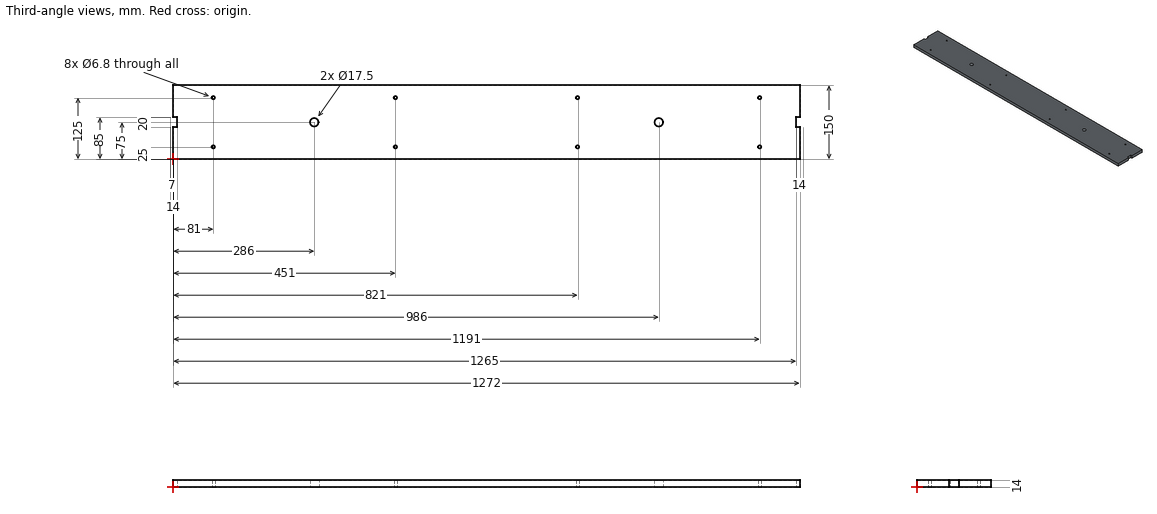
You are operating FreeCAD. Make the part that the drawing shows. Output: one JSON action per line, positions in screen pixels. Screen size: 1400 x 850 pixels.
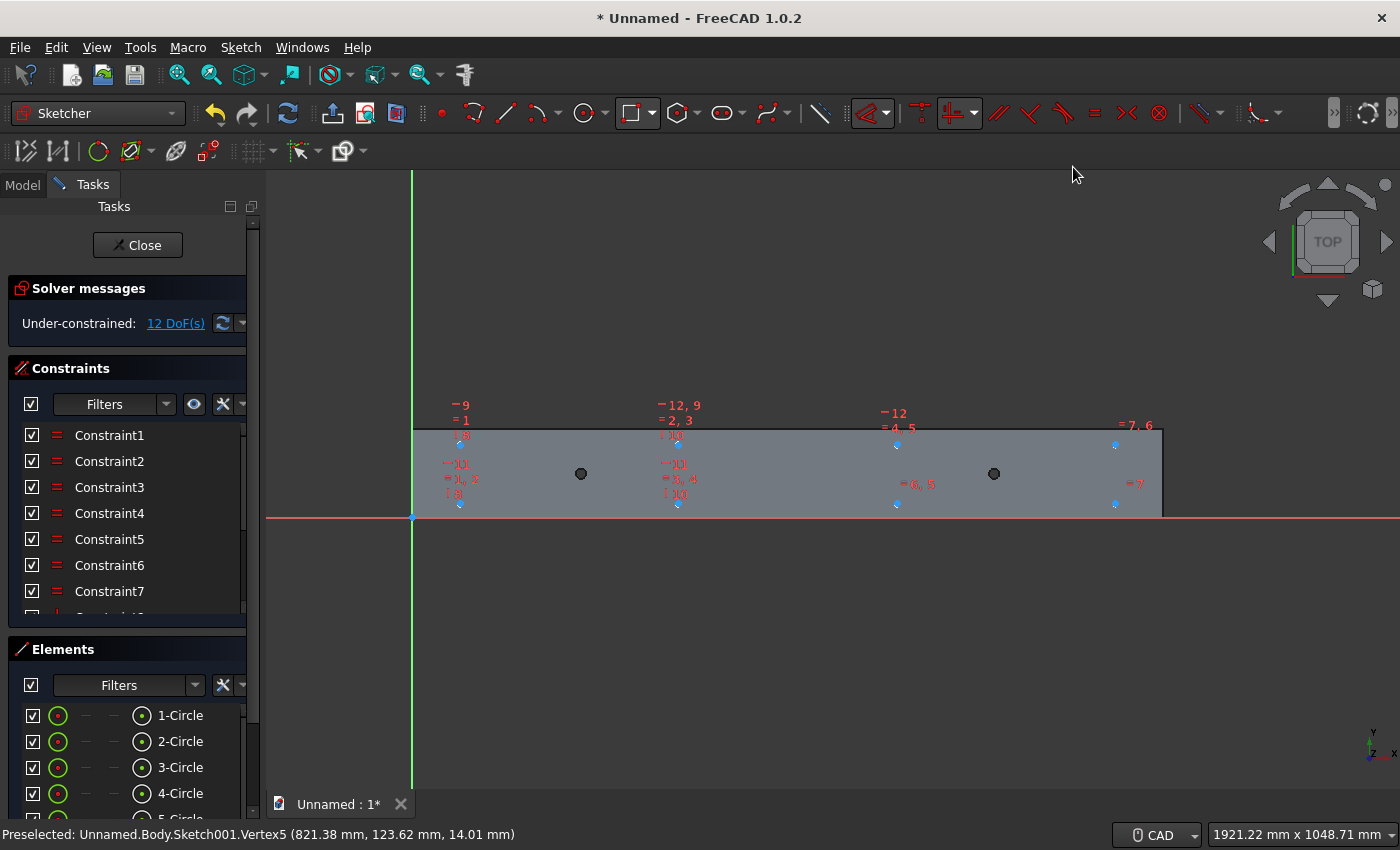
{"action": "left_click", "coordinate": [897, 445]}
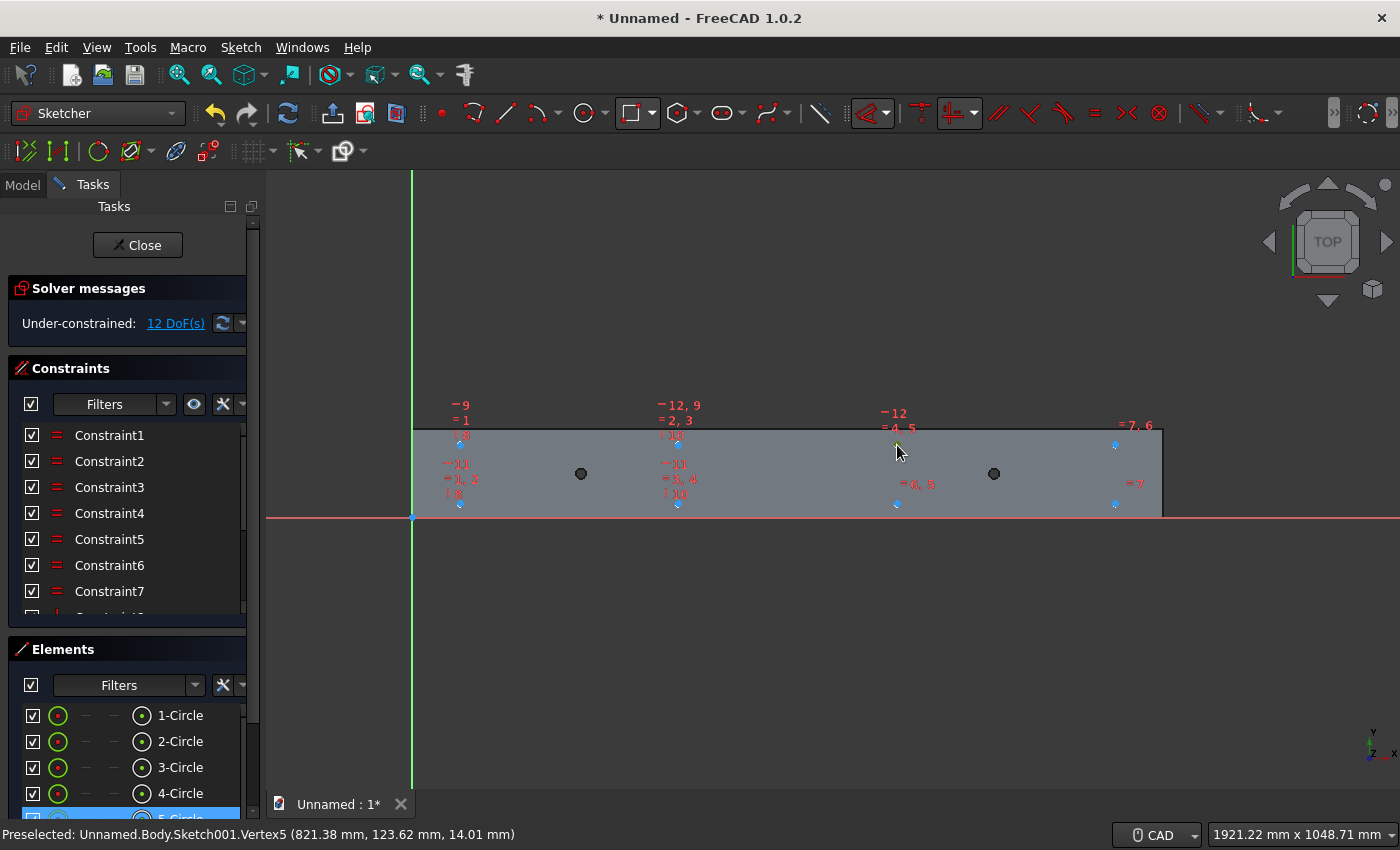
{"action": "left_click", "coordinate": [897, 504]}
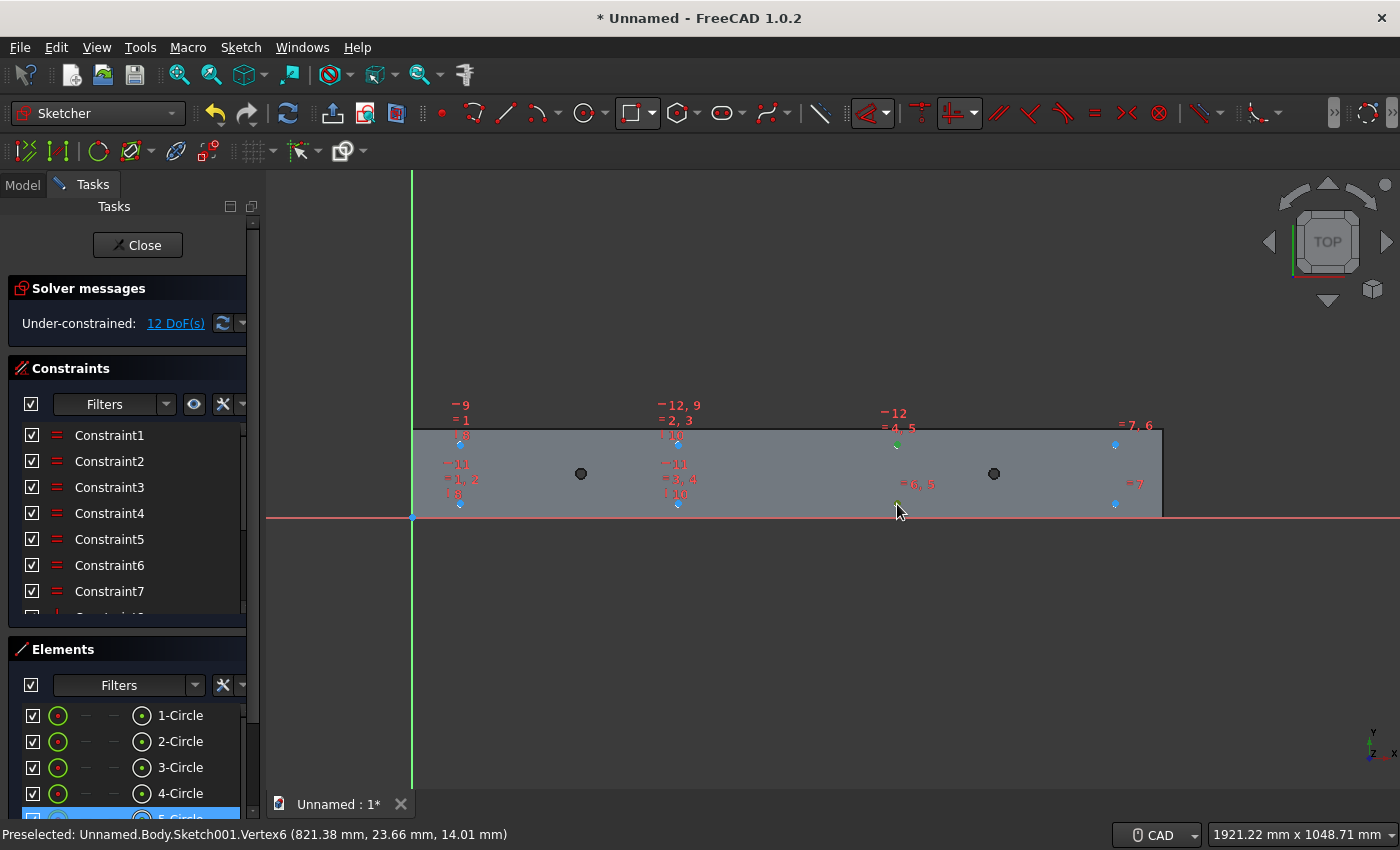
{"action": "key", "text": "v"}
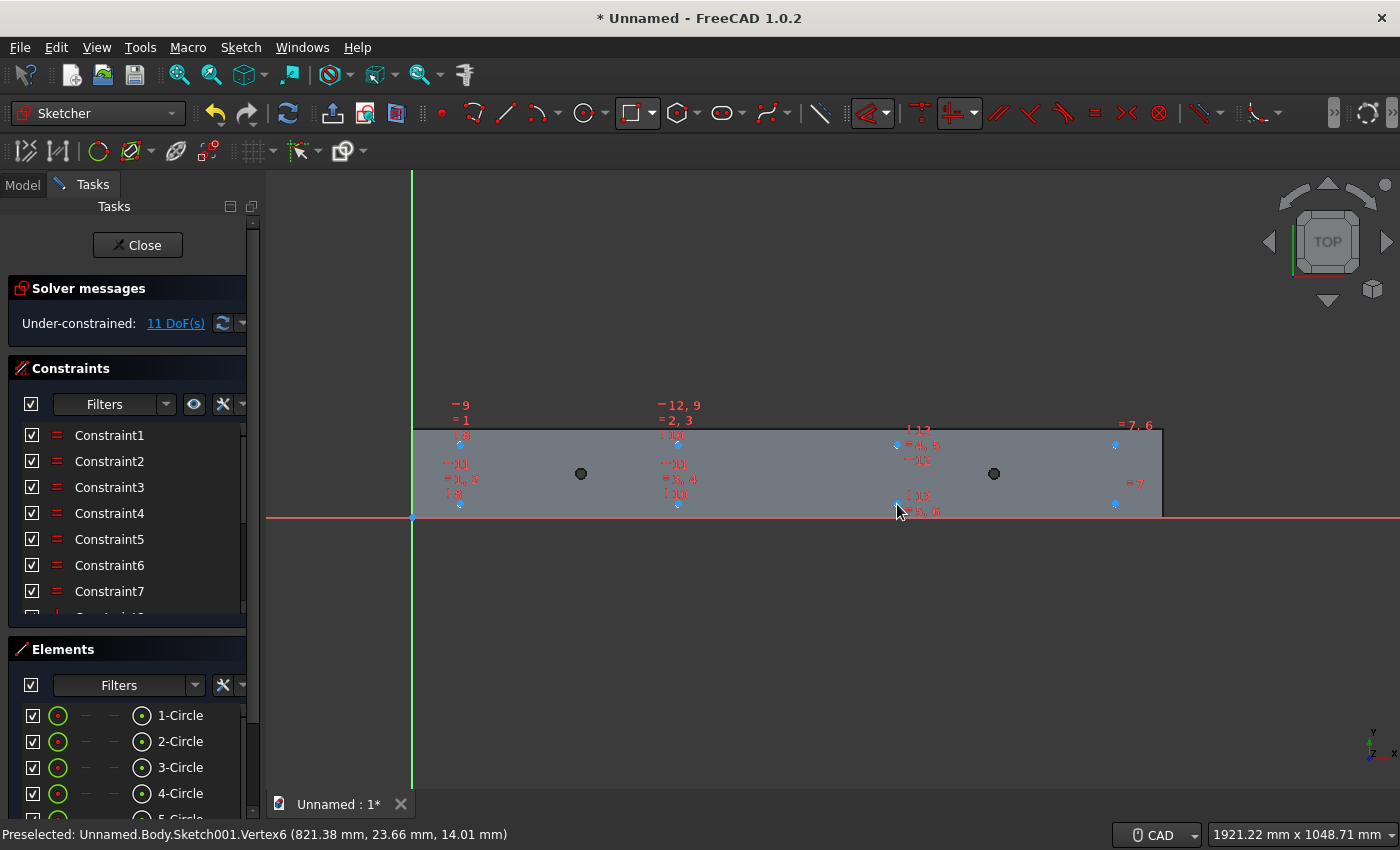
{"action": "left_click", "coordinate": [678, 504]}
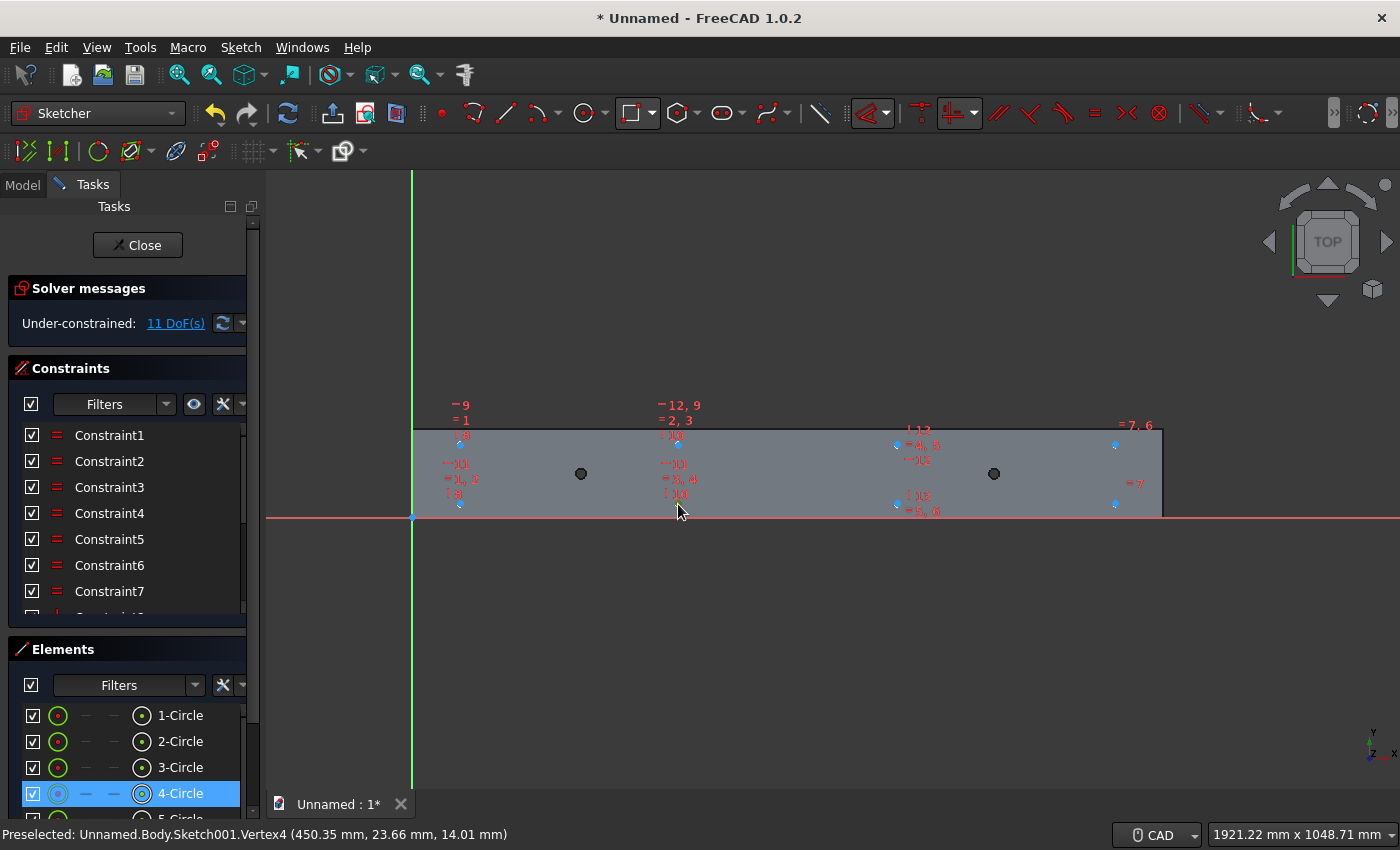
{"action": "left_click", "coordinate": [897, 504]}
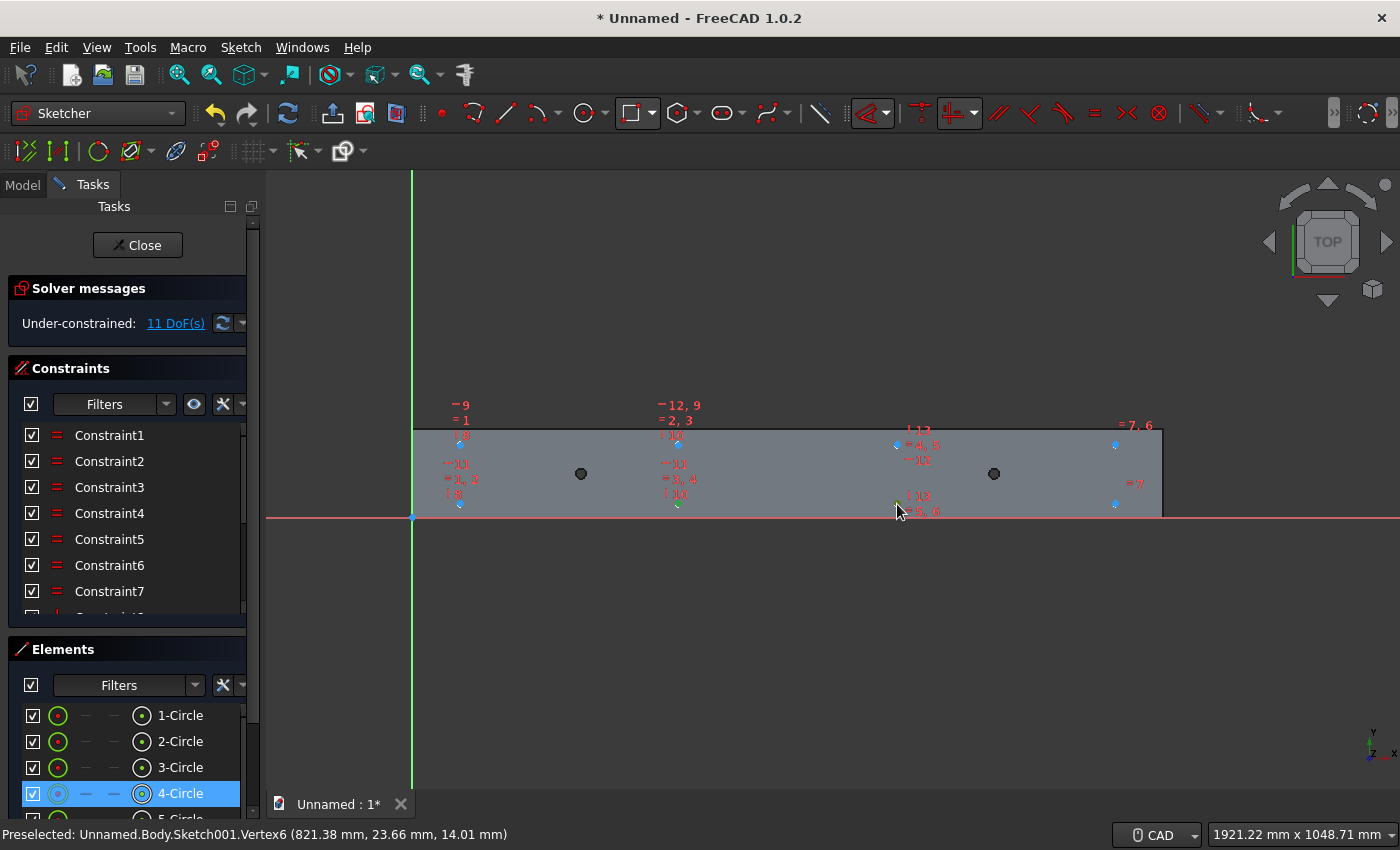
{"action": "left_click", "coordinate": [976, 114]}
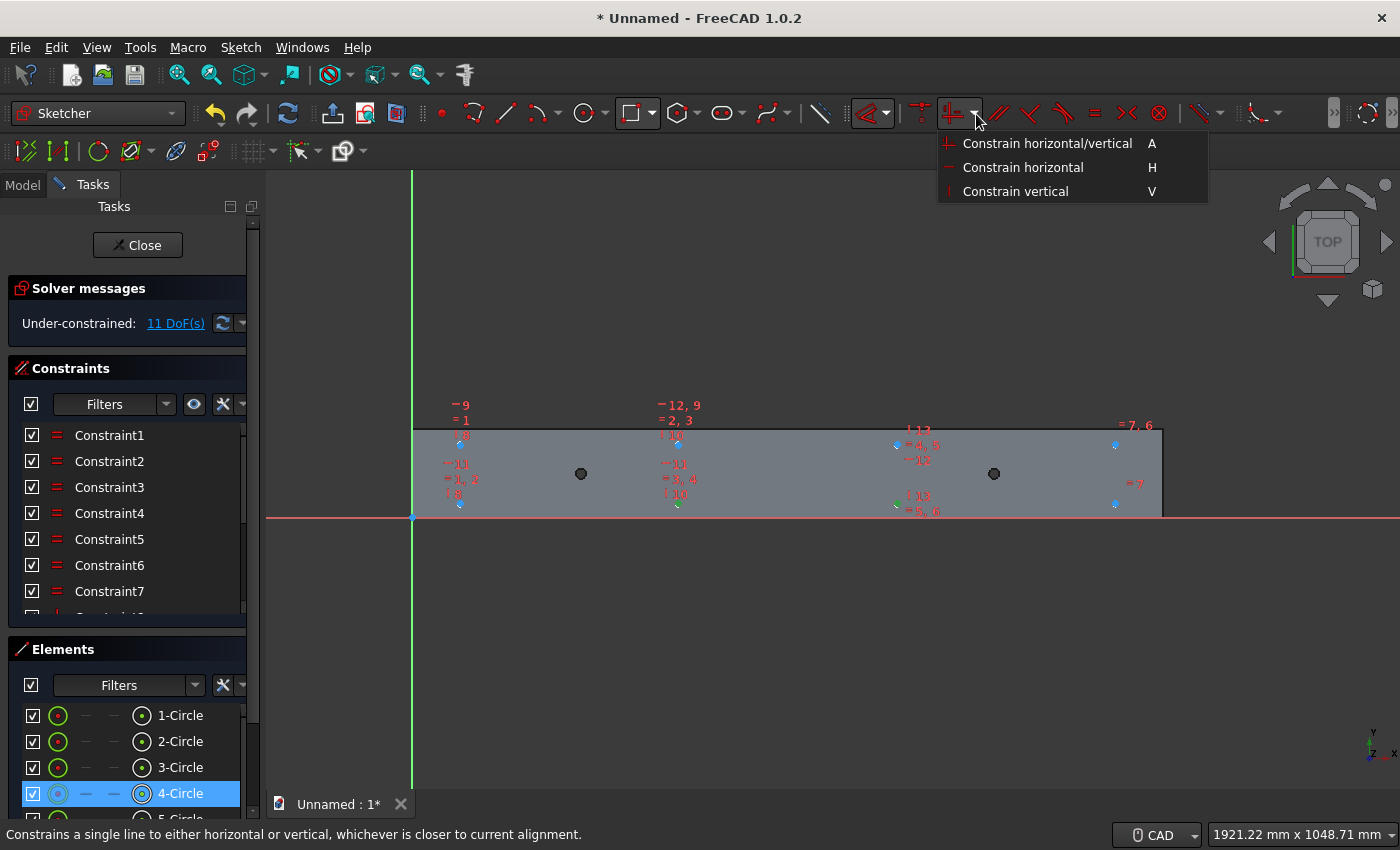
{"action": "left_click", "coordinate": [1073, 167]}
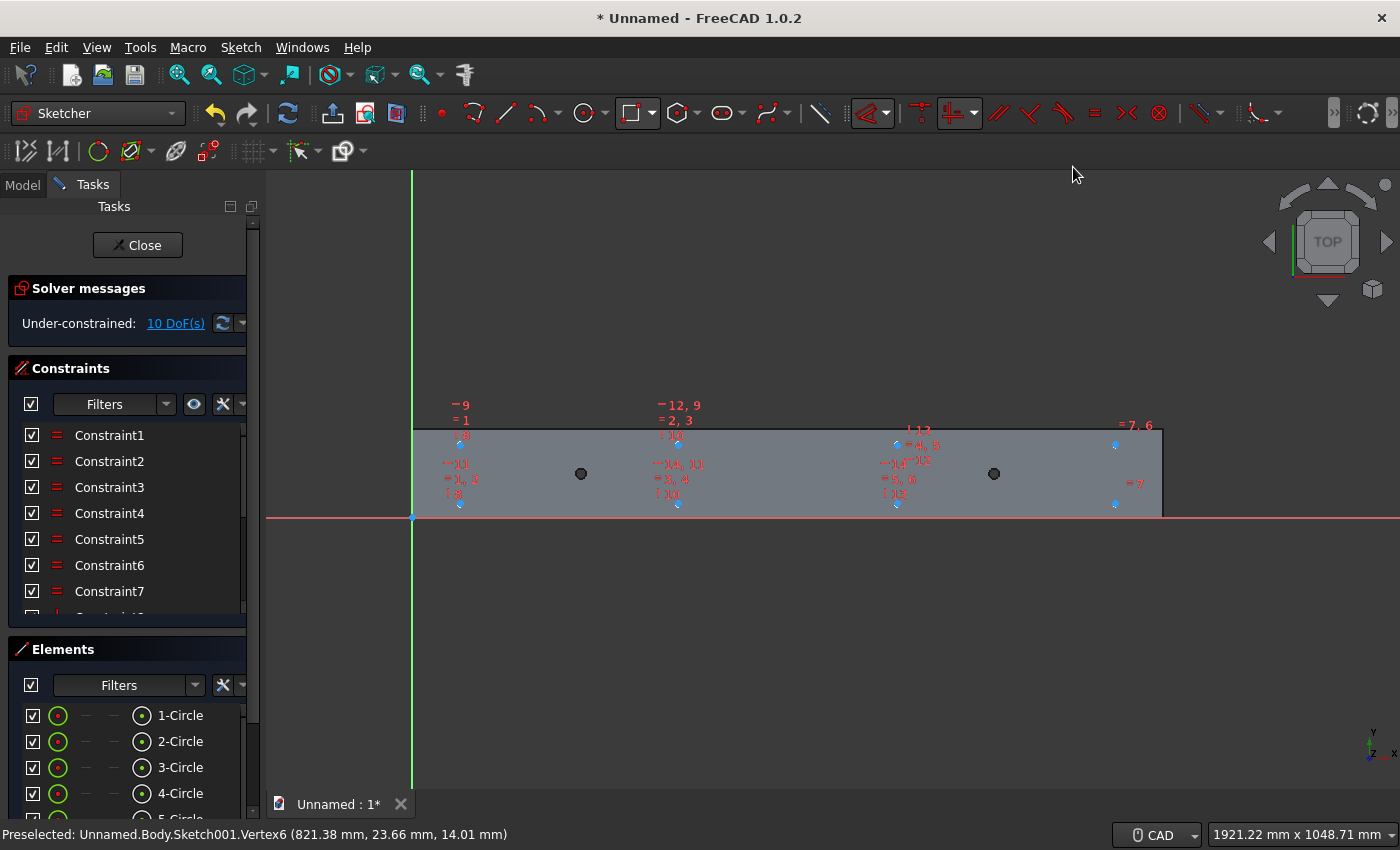
{"action": "left_click", "coordinate": [897, 445]}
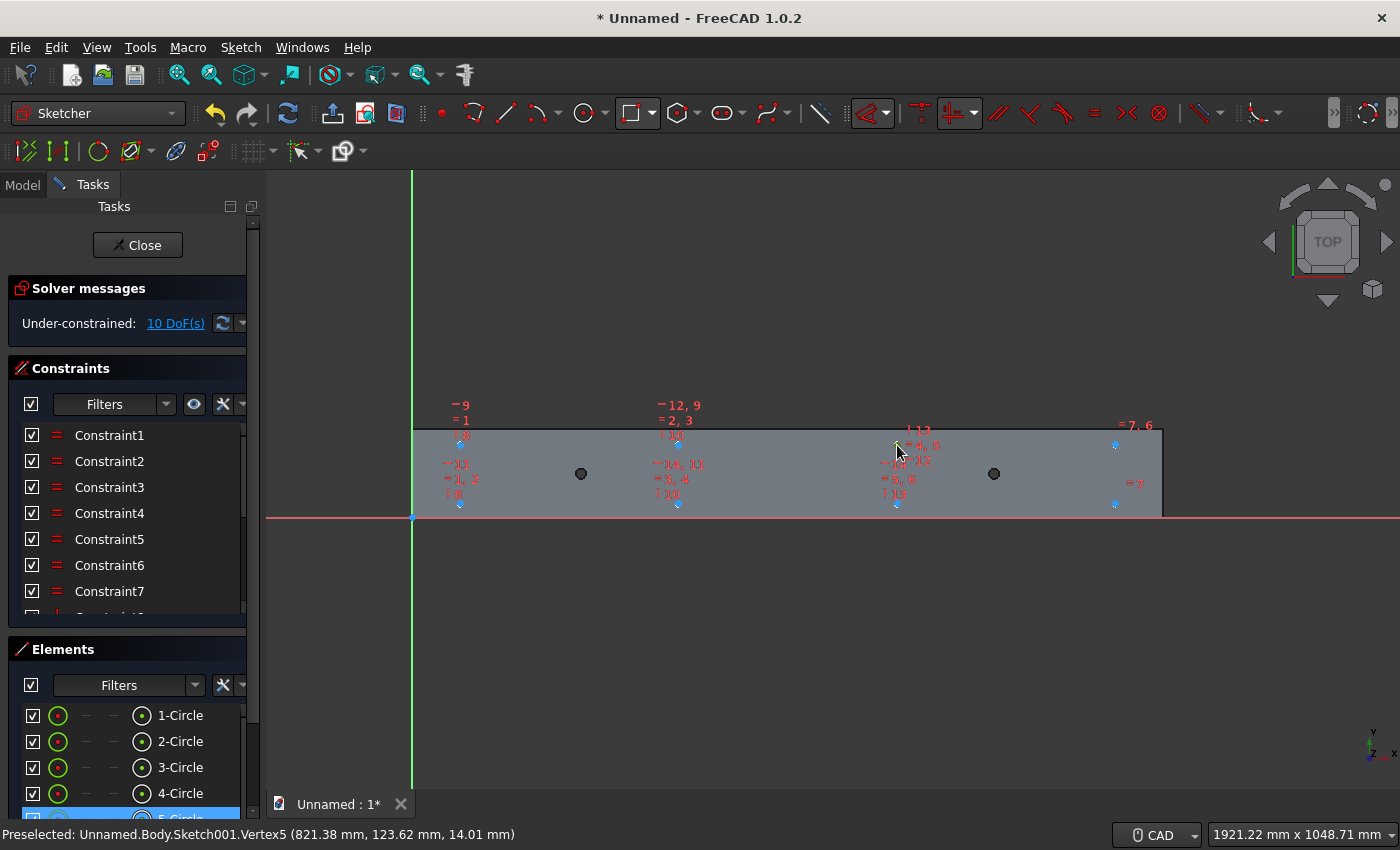
{"action": "left_click", "coordinate": [1115, 445]}